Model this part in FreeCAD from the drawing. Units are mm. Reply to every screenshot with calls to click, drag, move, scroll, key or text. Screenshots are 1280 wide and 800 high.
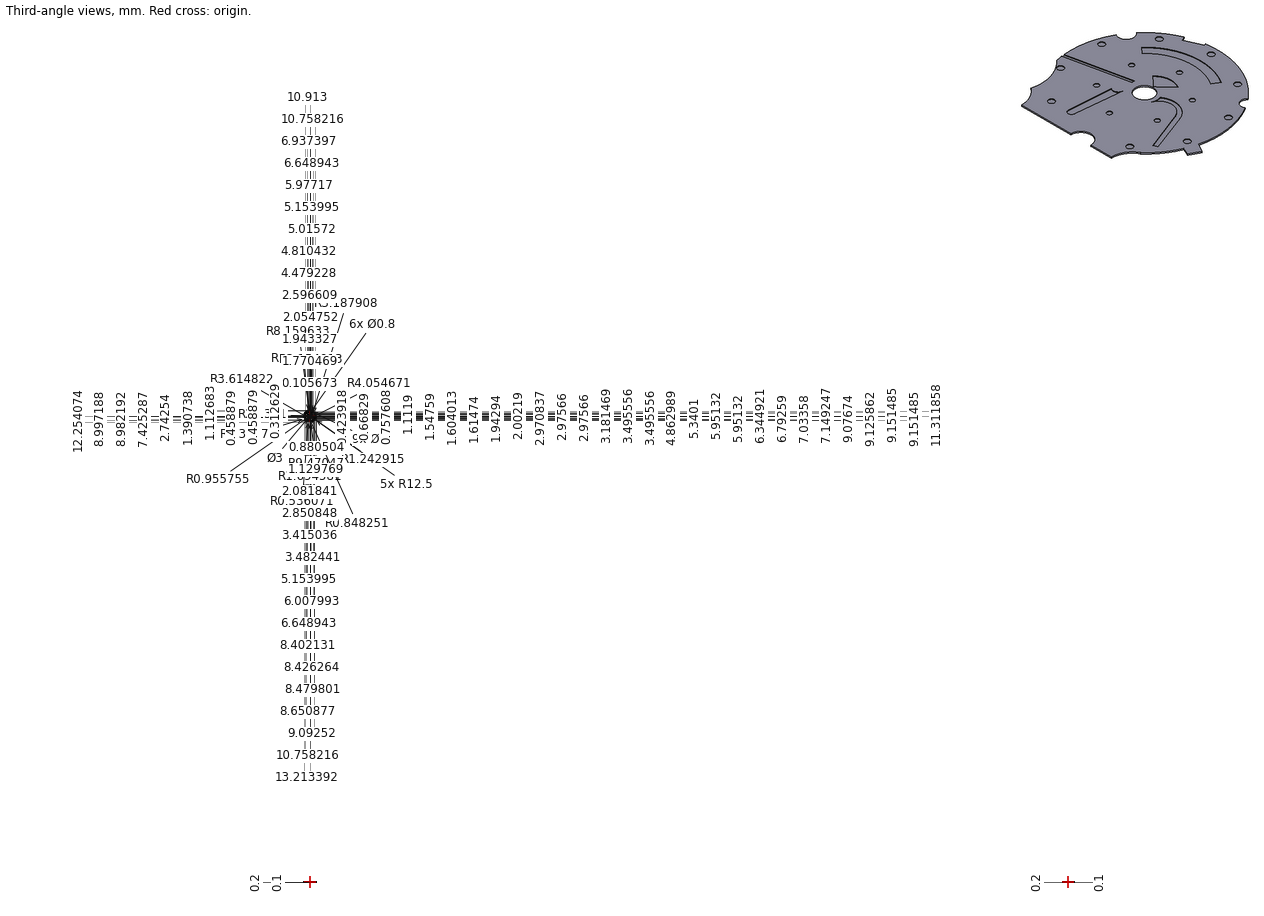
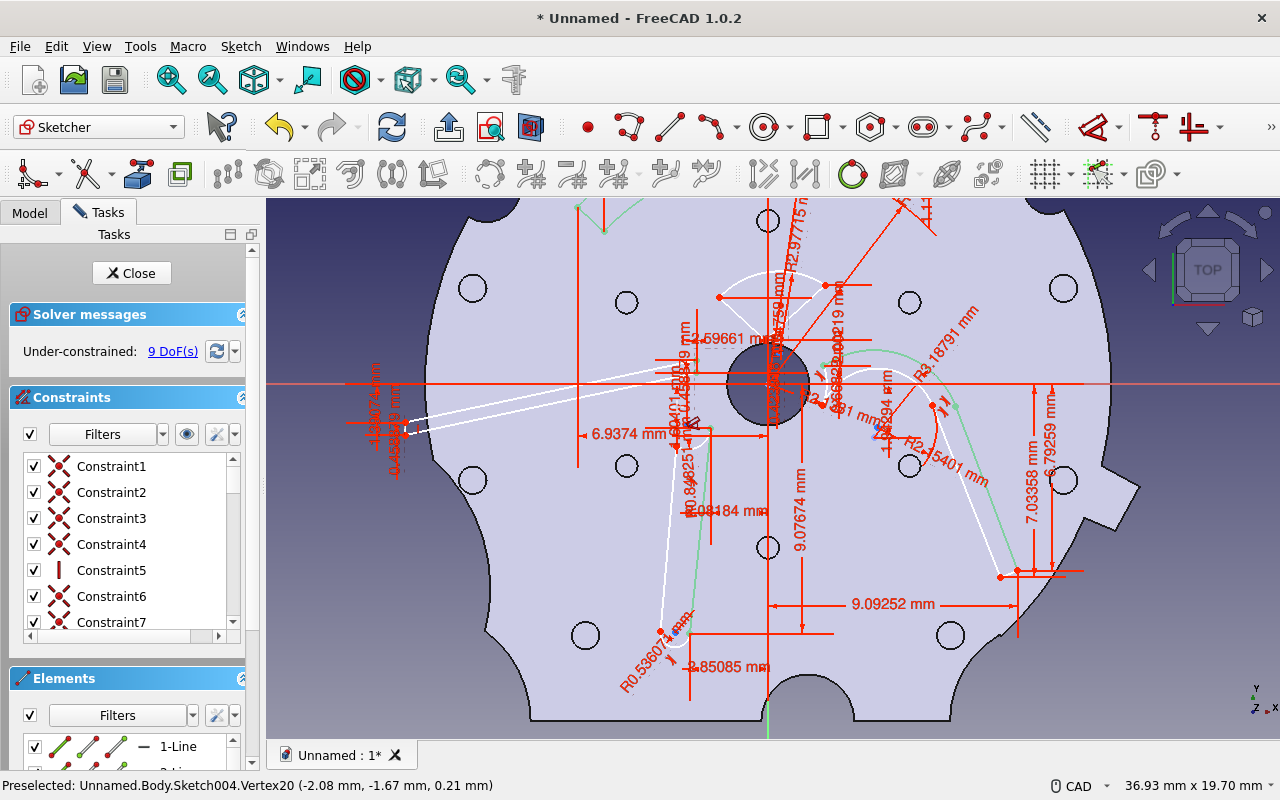
click(676, 446)
click(701, 302)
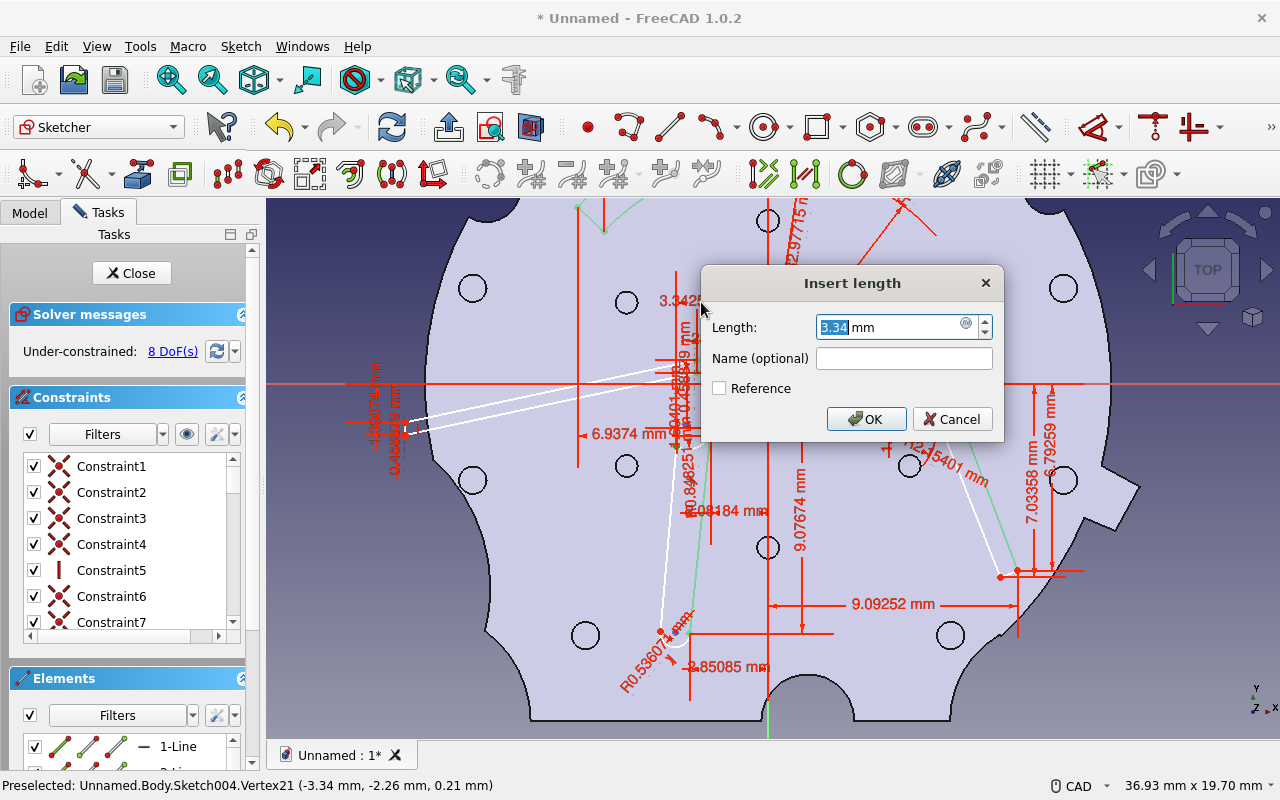
text(3.415036)
key(Return)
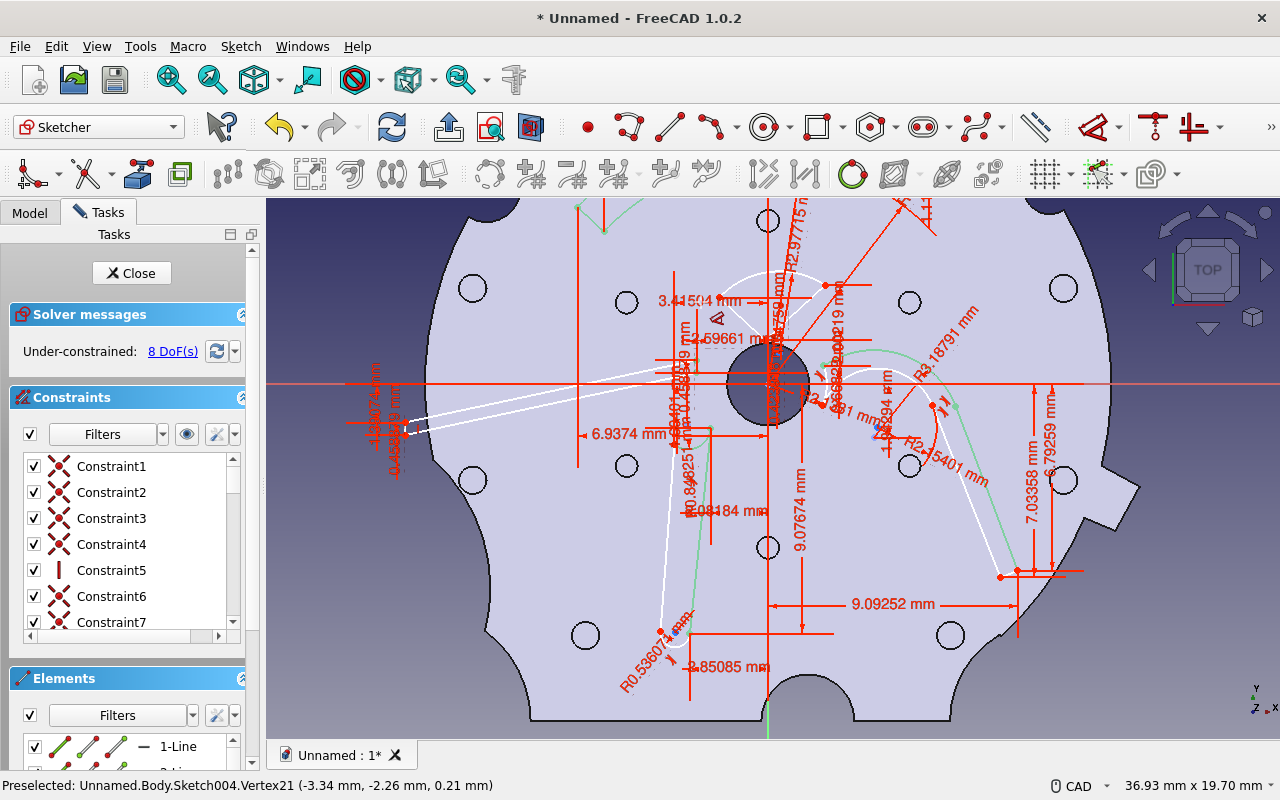
click(661, 632)
click(802, 451)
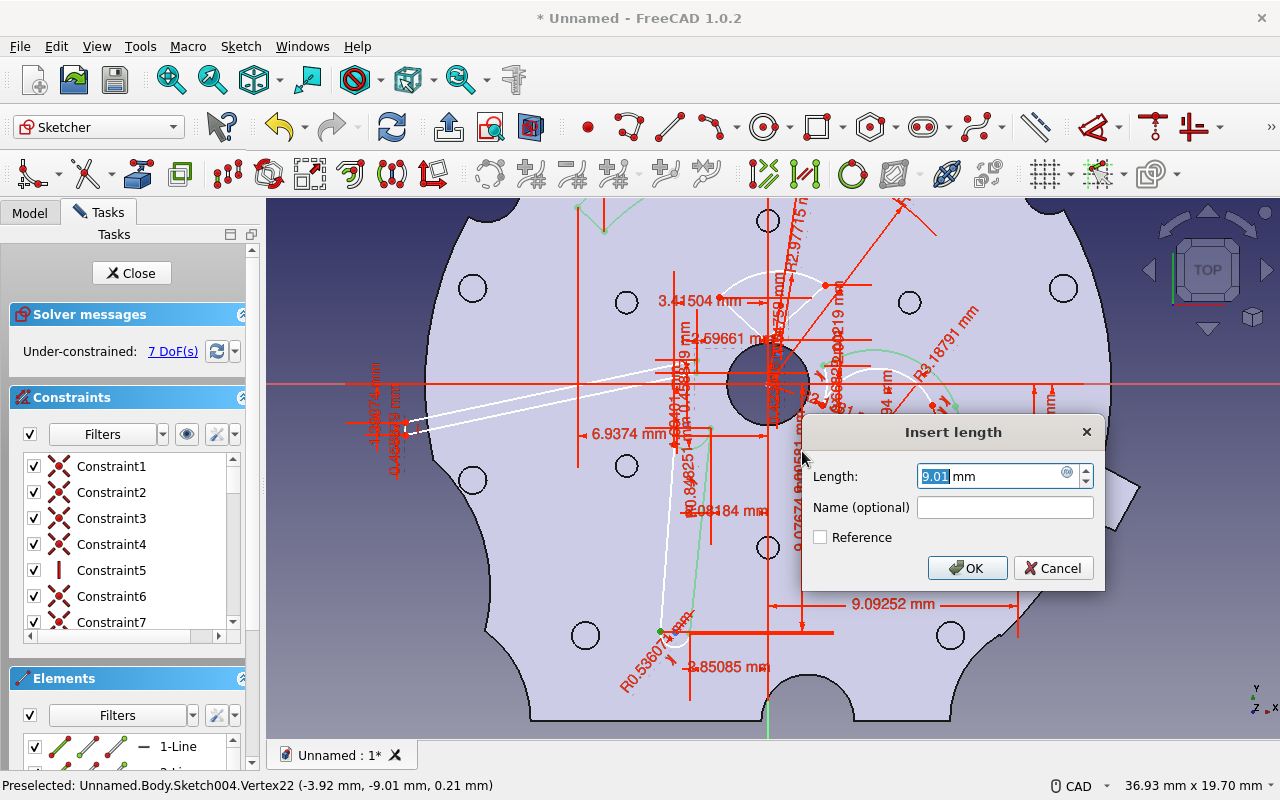
text(8.997188)
key(Return)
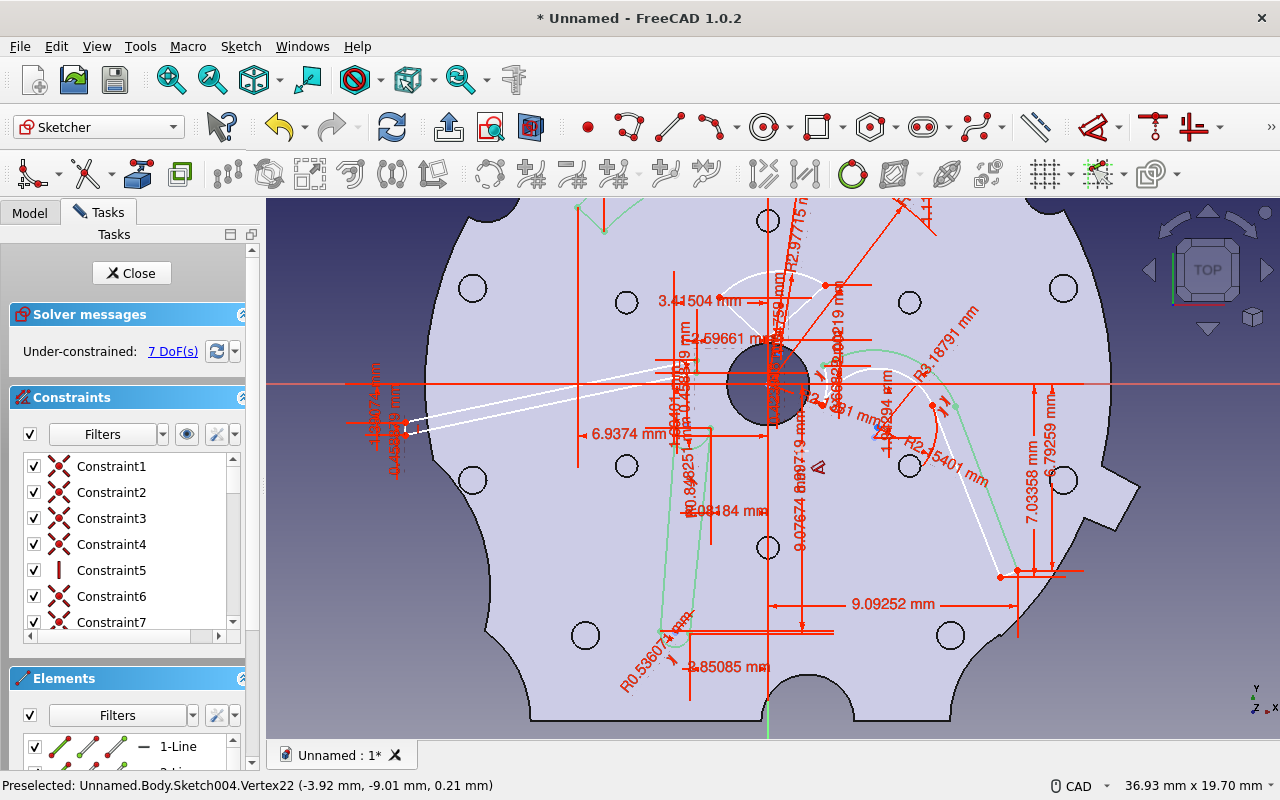
click(719, 298)
click(744, 264)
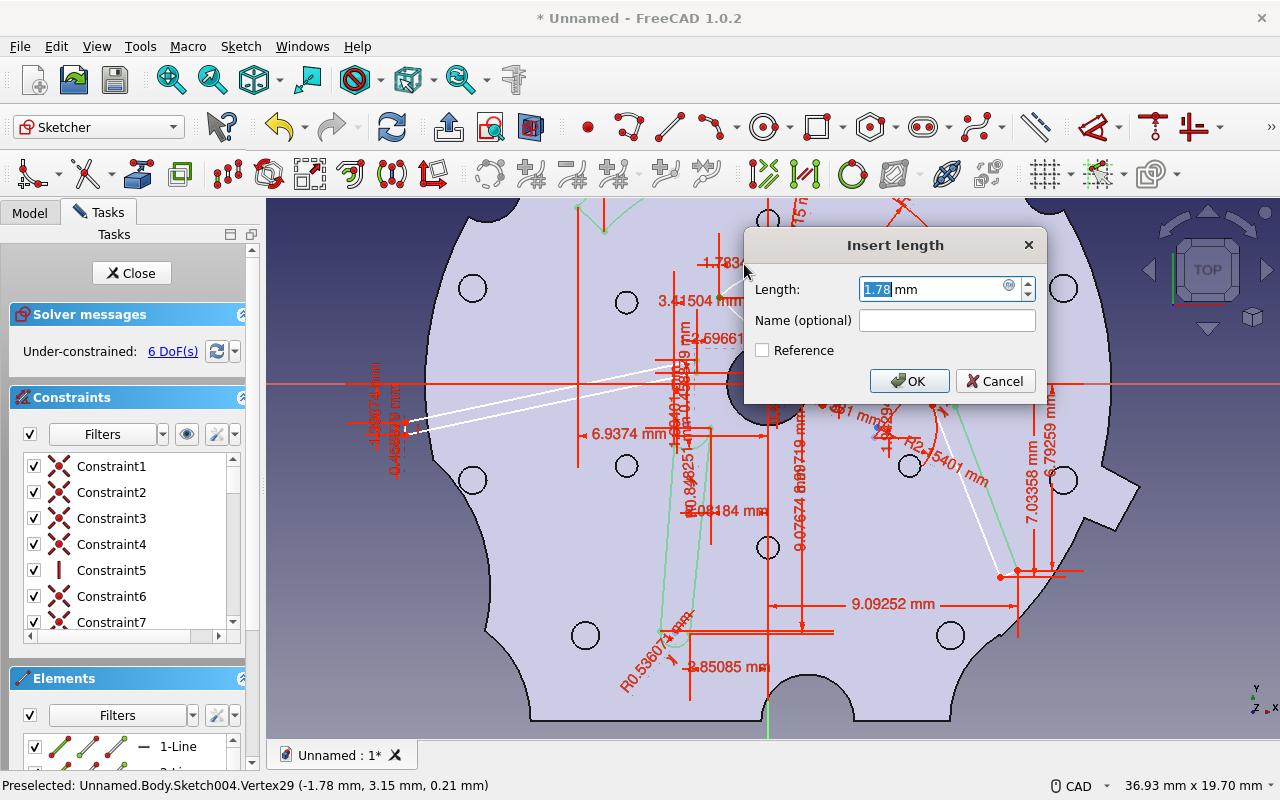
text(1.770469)
key(Return)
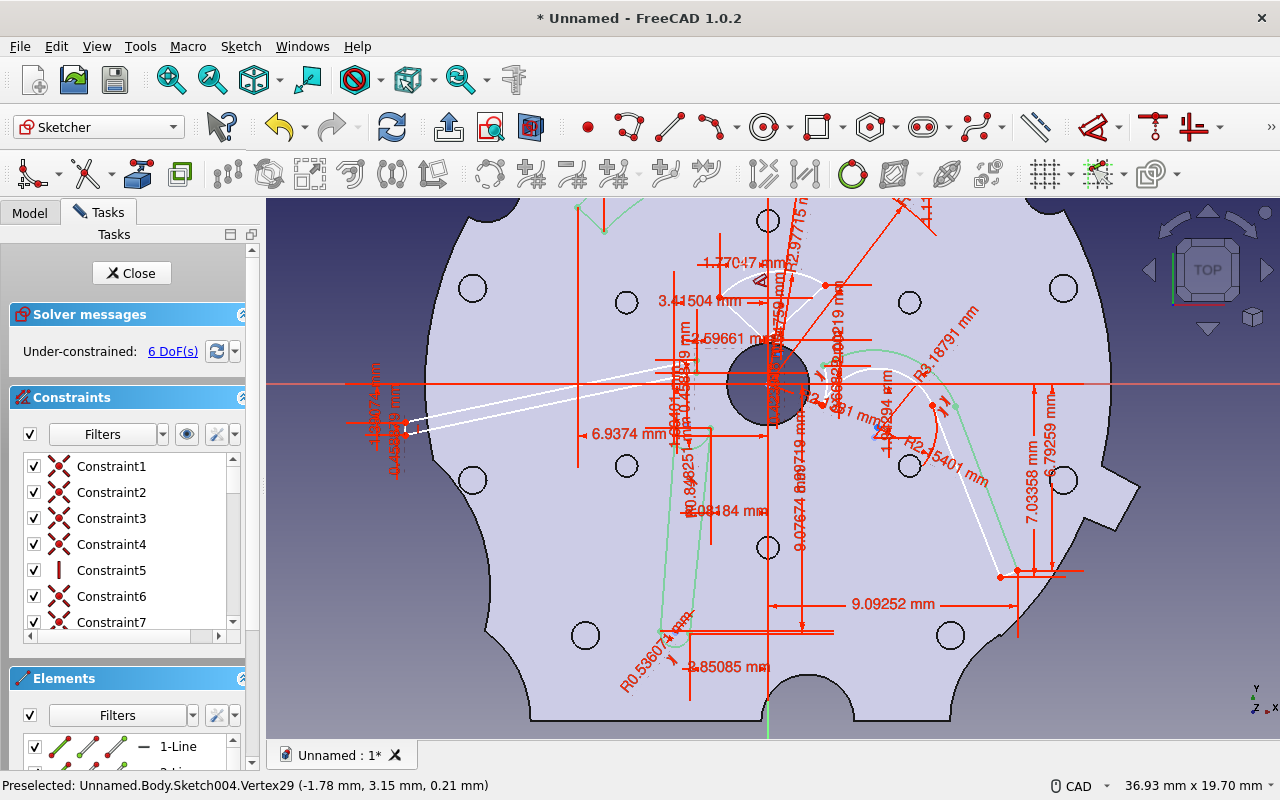
click(720, 298)
click(662, 341)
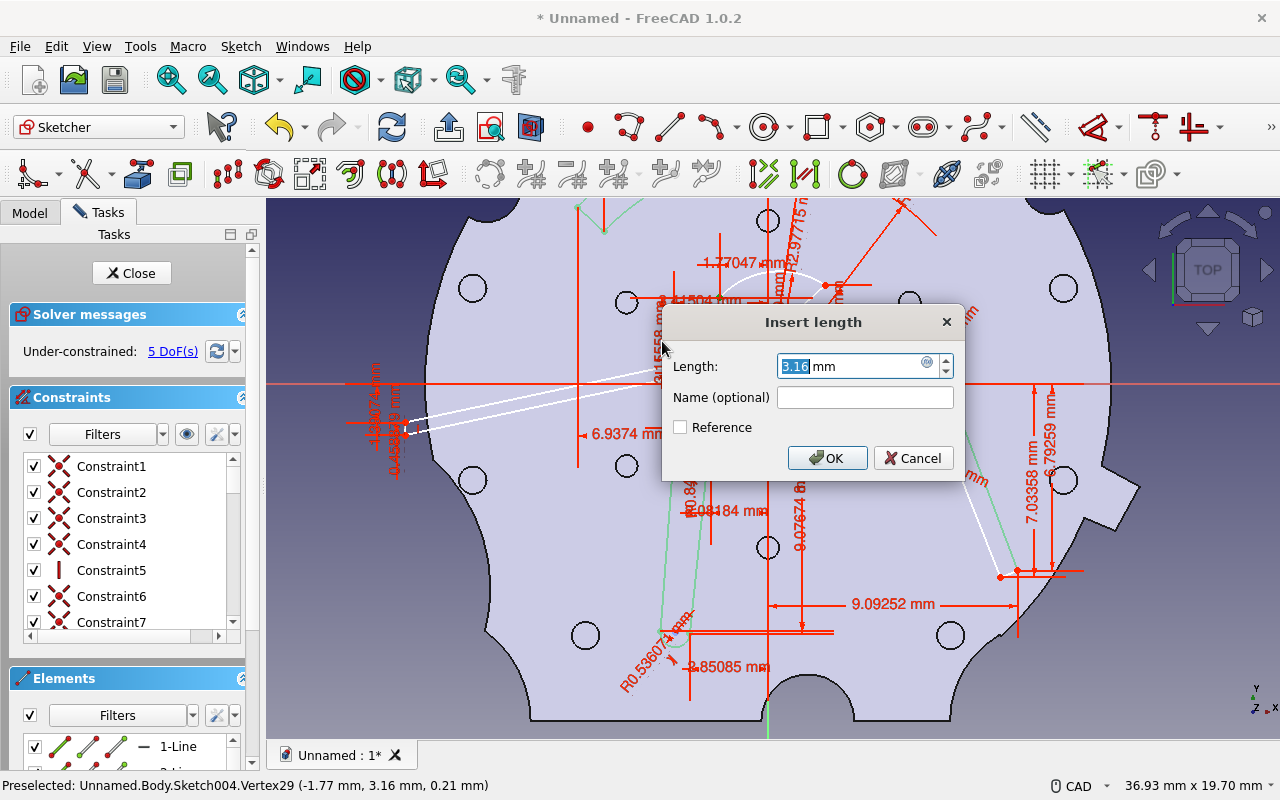
text(3.181469)
key(Return)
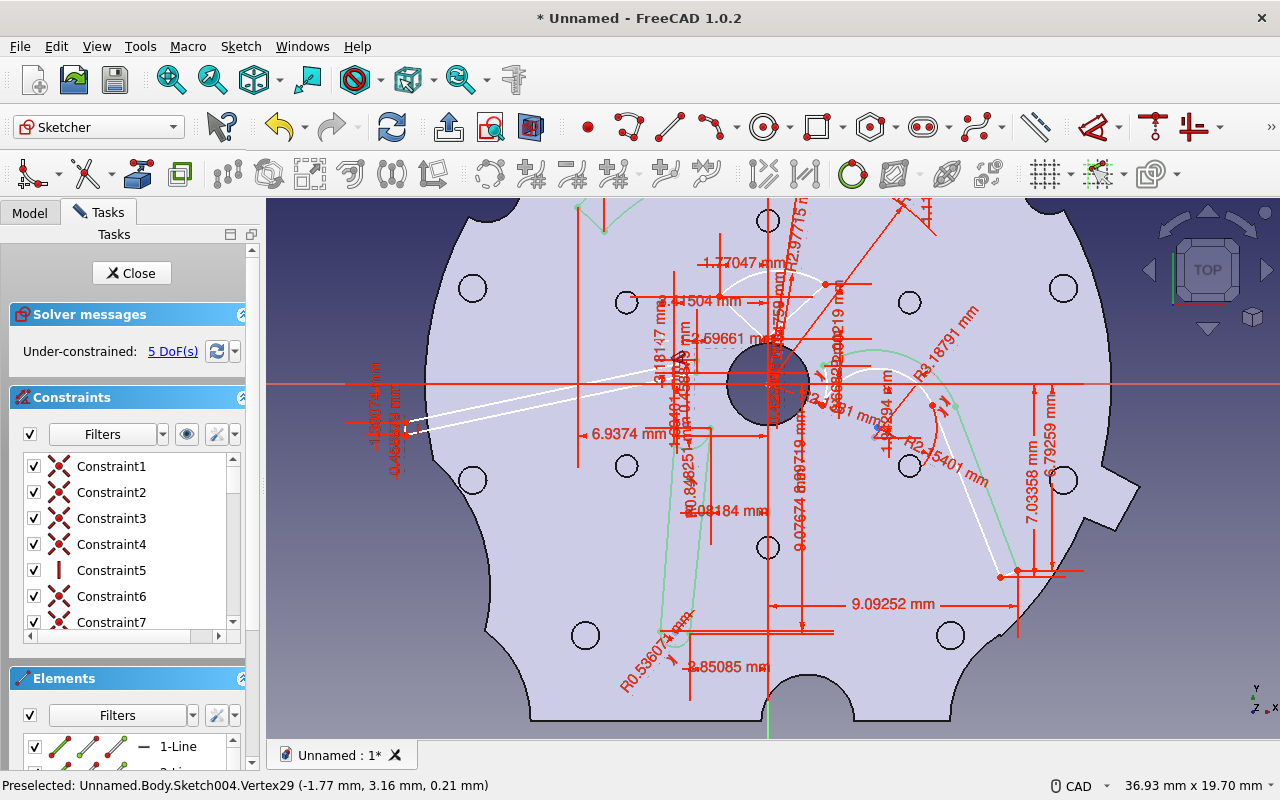
scroll(765, 339, up, 14)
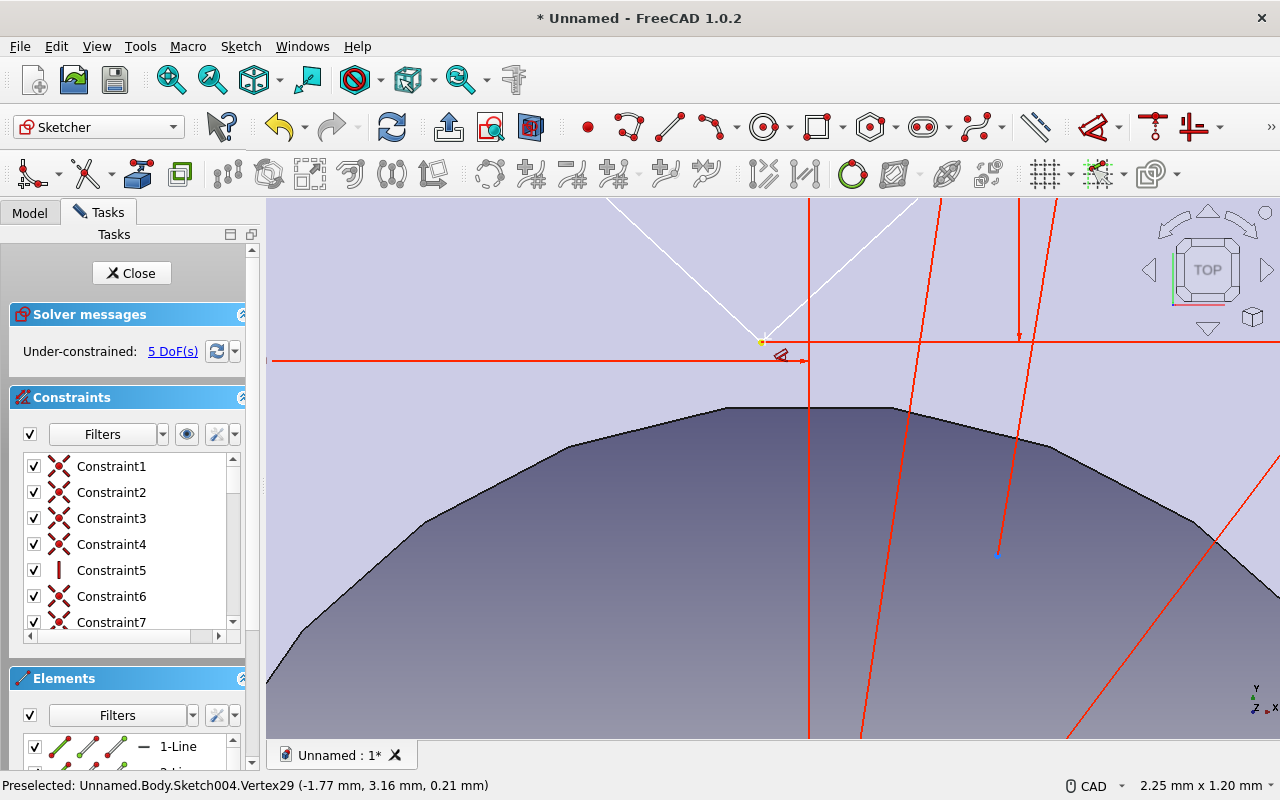
click(761, 342)
click(774, 308)